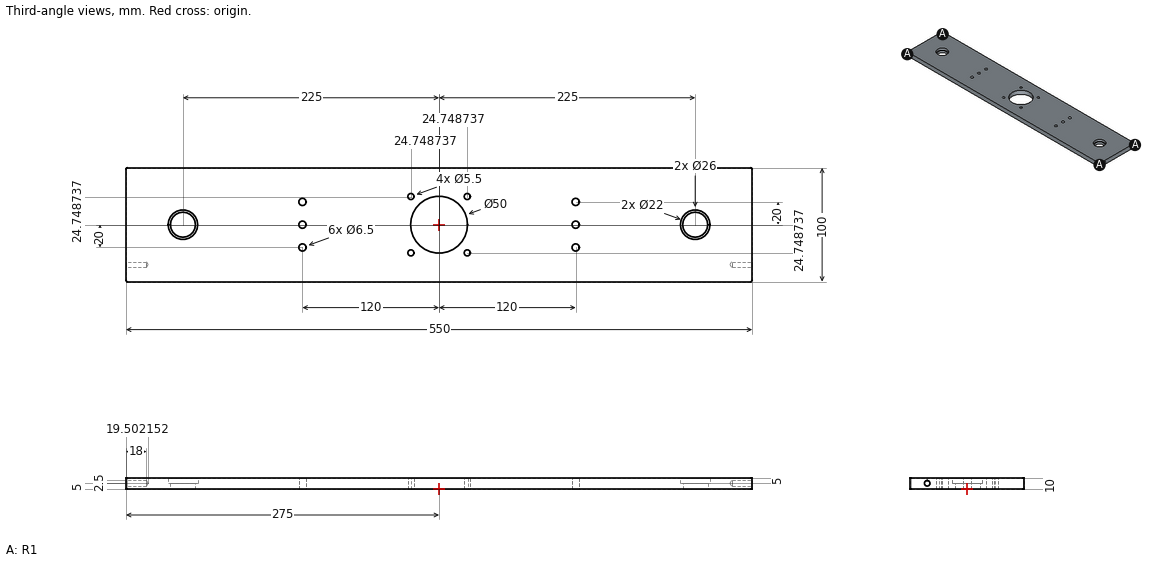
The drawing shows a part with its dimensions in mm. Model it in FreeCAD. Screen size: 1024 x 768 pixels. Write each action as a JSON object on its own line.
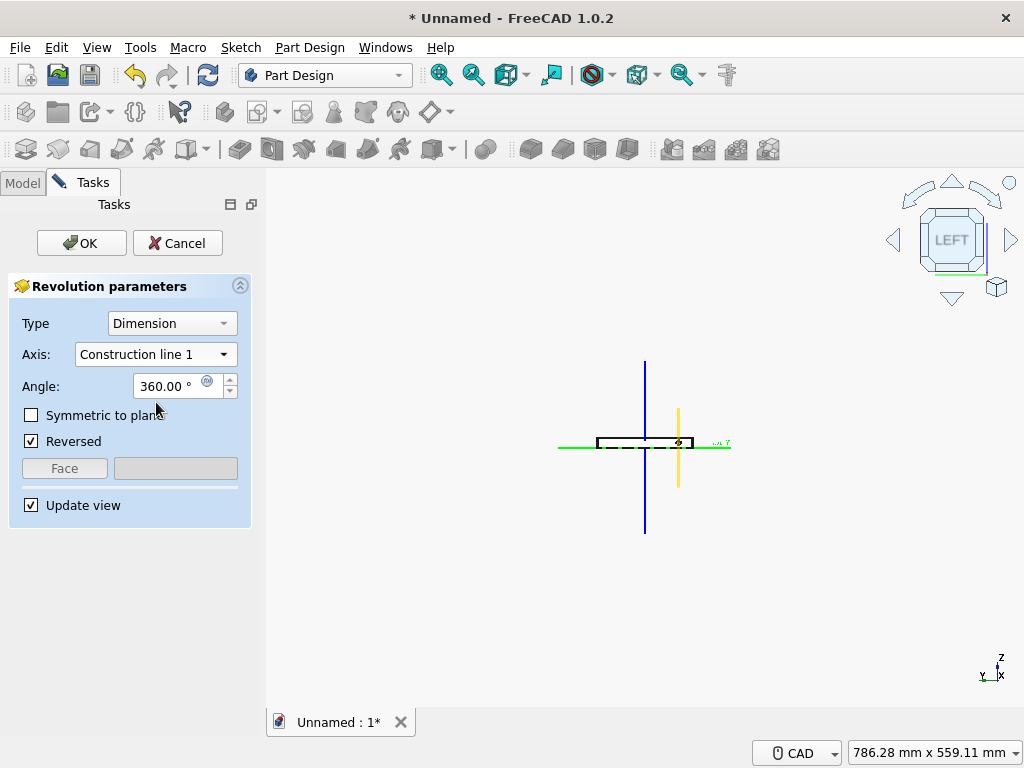
{"action": "left_click", "coordinate": [82, 243]}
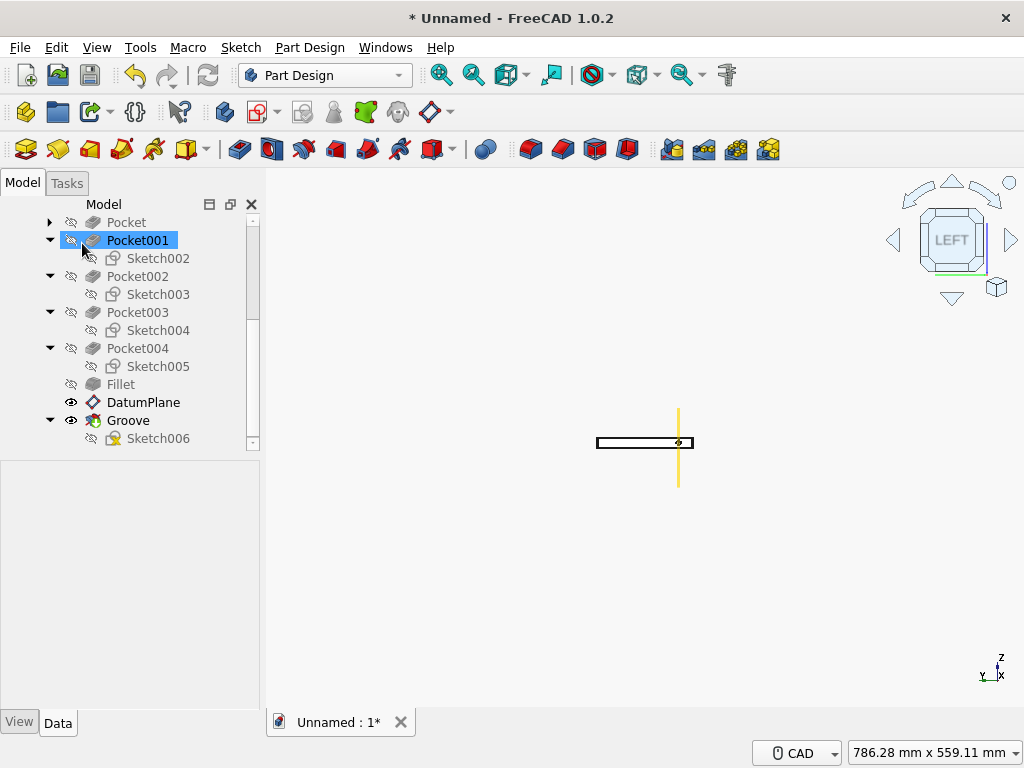
{"action": "left_click", "coordinate": [116, 402]}
{"action": "key", "text": "space"}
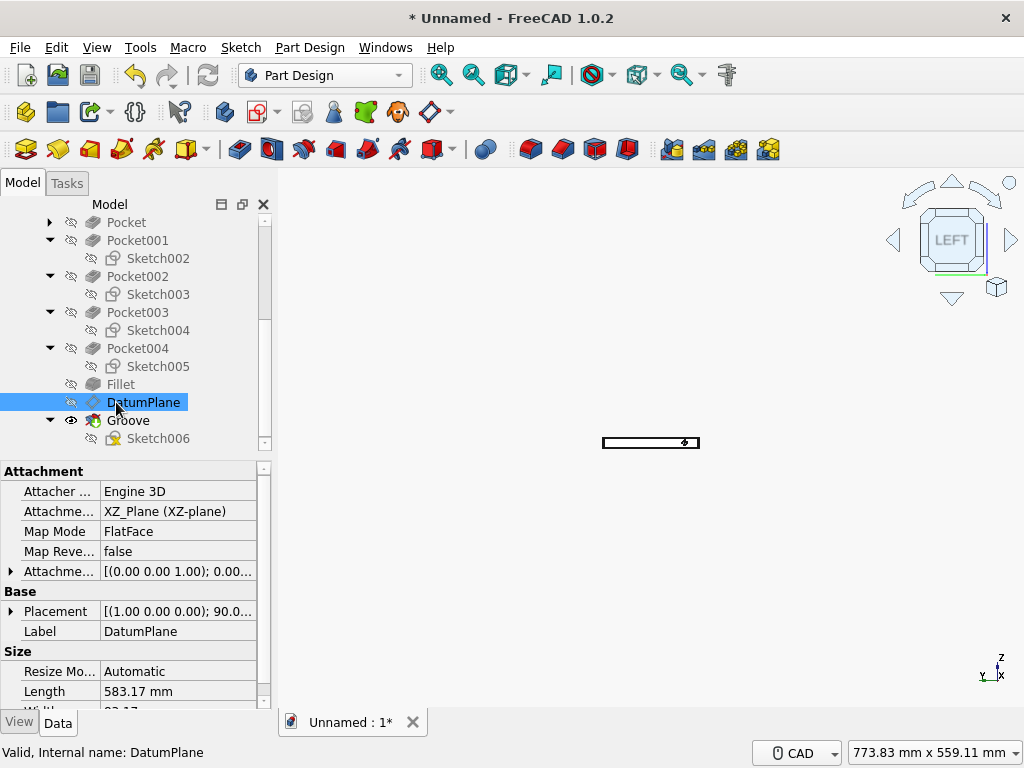
{"action": "key", "text": "v f"}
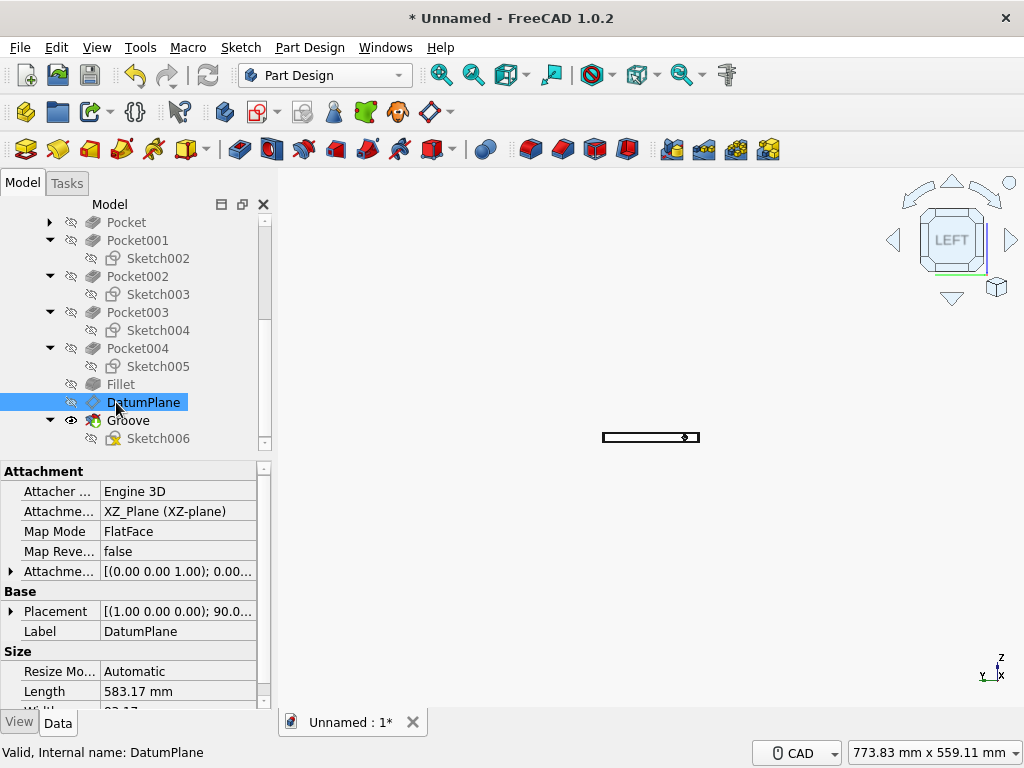
{"action": "left_click", "coordinate": [116, 420]}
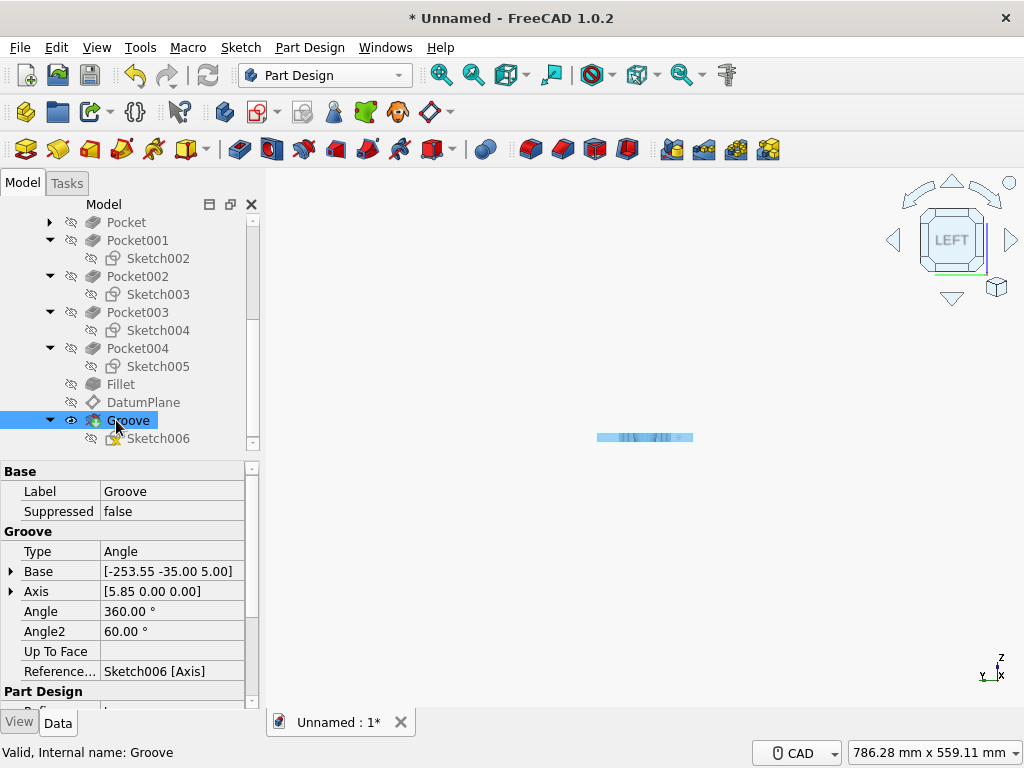
{"action": "left_click", "coordinate": [672, 150]}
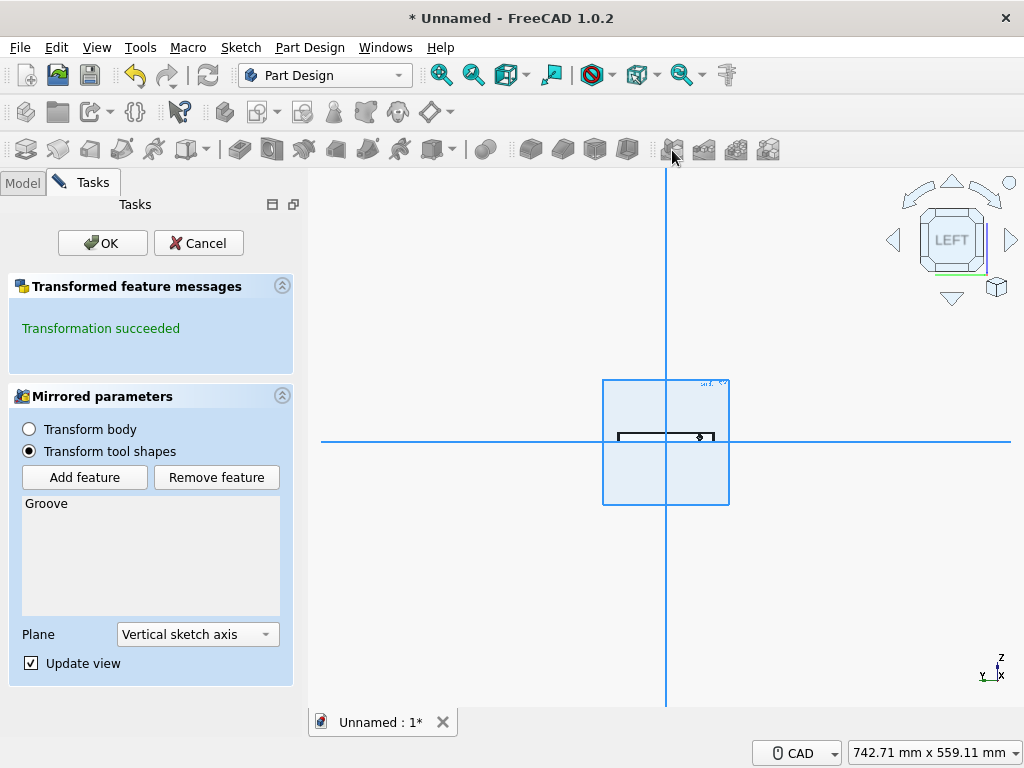
{"action": "left_click", "coordinate": [198, 634]}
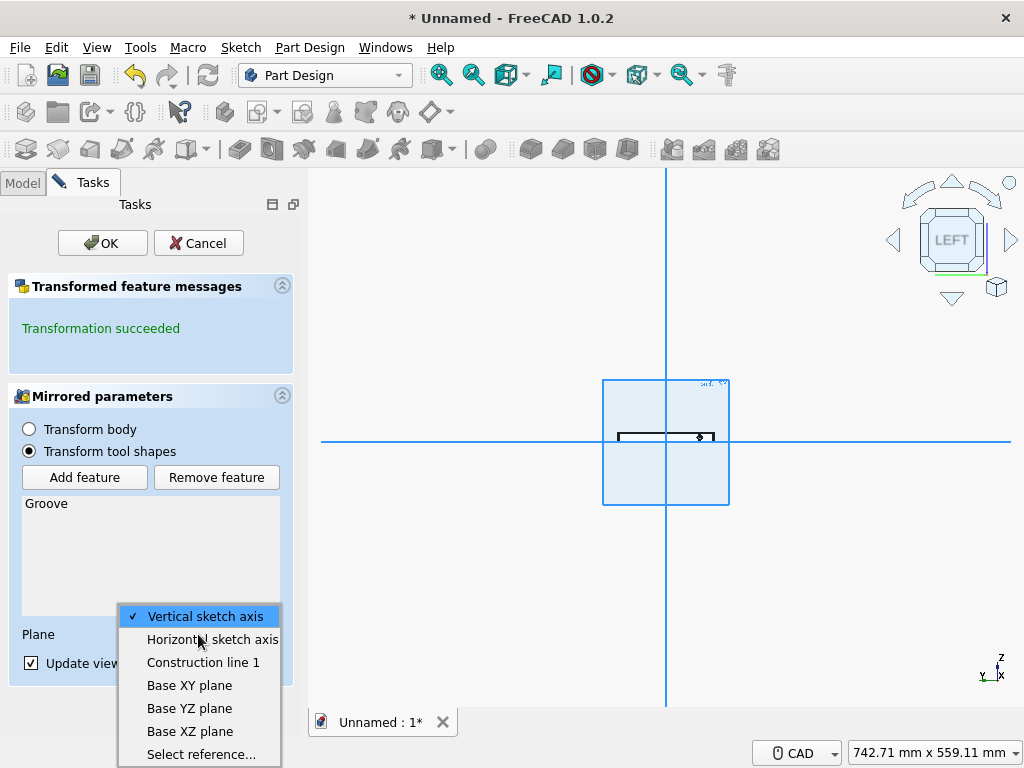
{"action": "left_click", "coordinate": [198, 708]}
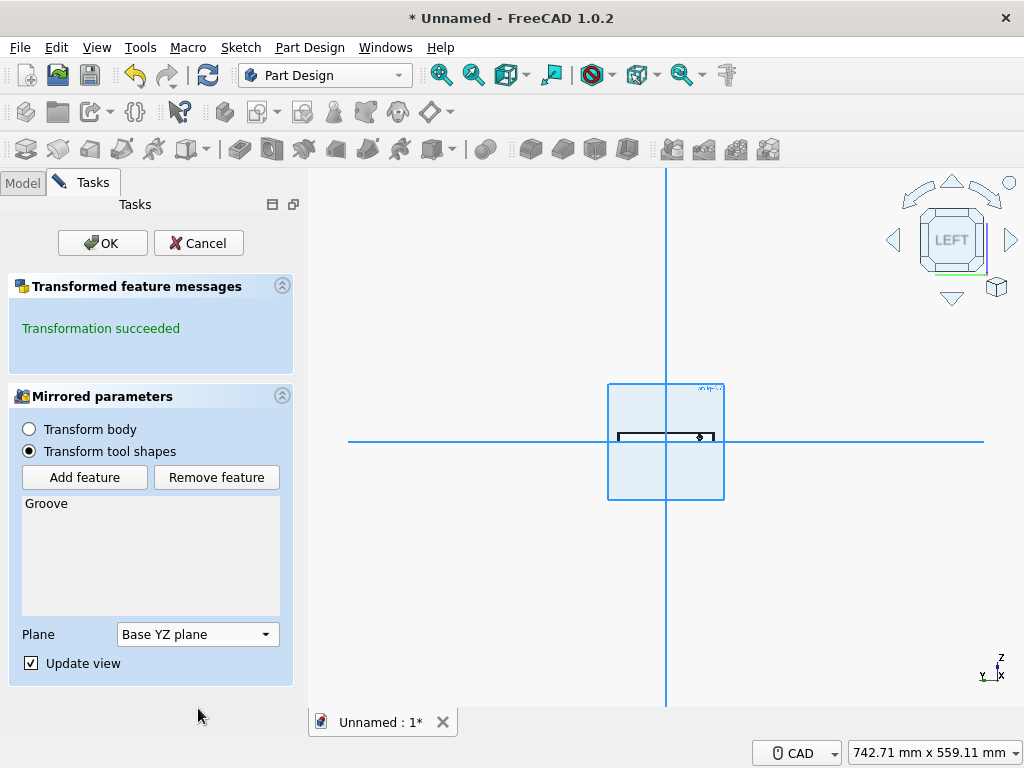
{"action": "left_click", "coordinate": [103, 243]}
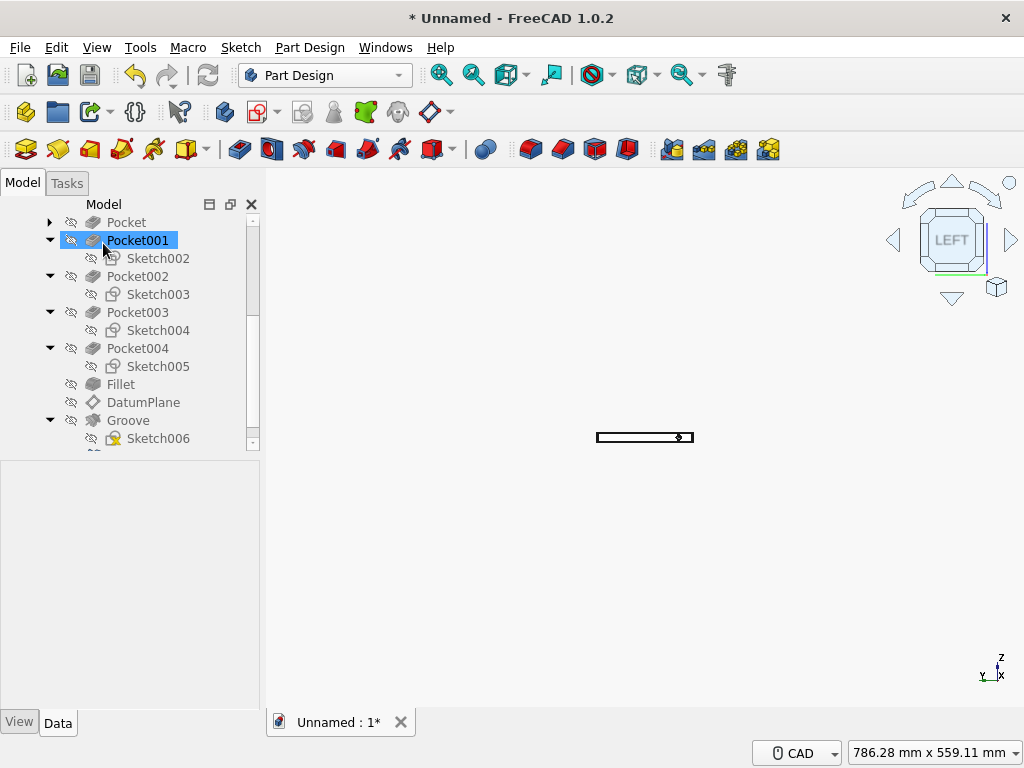
{"action": "key", "text": "0"}